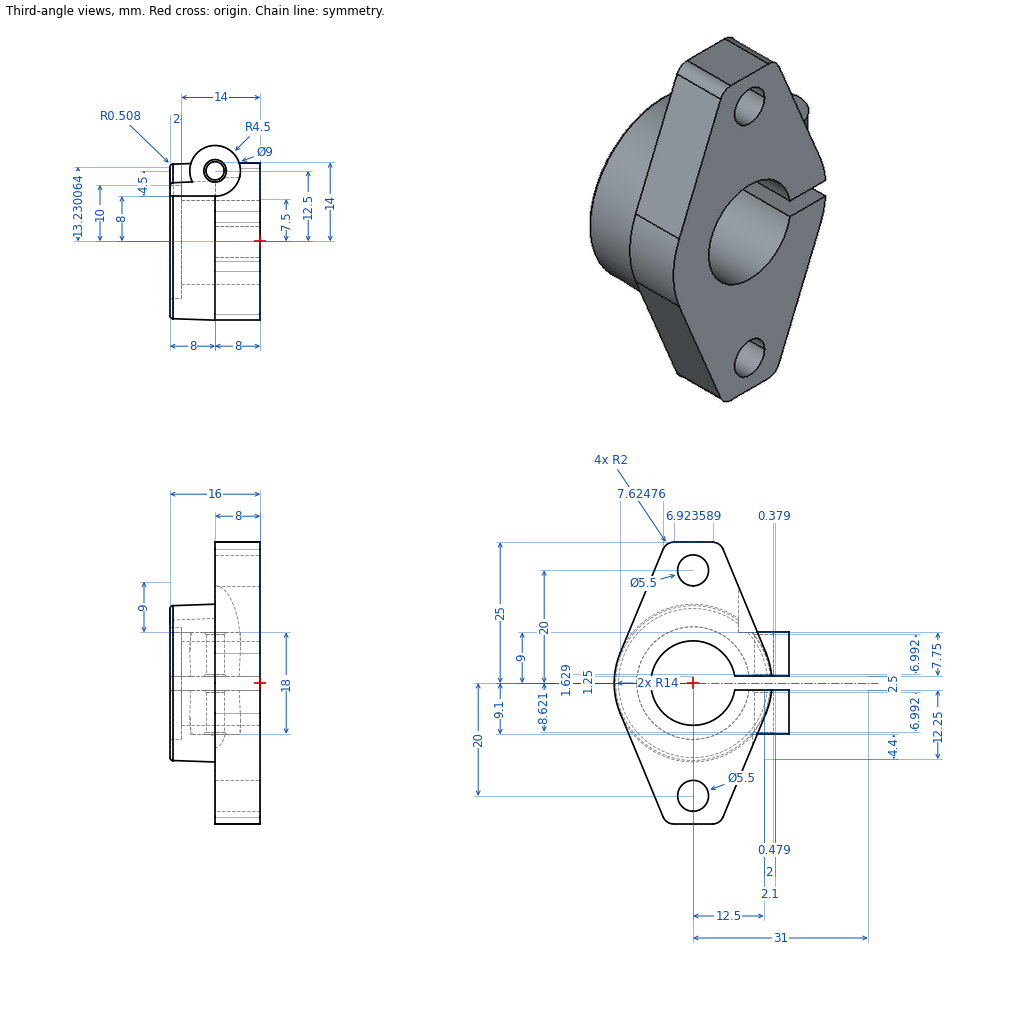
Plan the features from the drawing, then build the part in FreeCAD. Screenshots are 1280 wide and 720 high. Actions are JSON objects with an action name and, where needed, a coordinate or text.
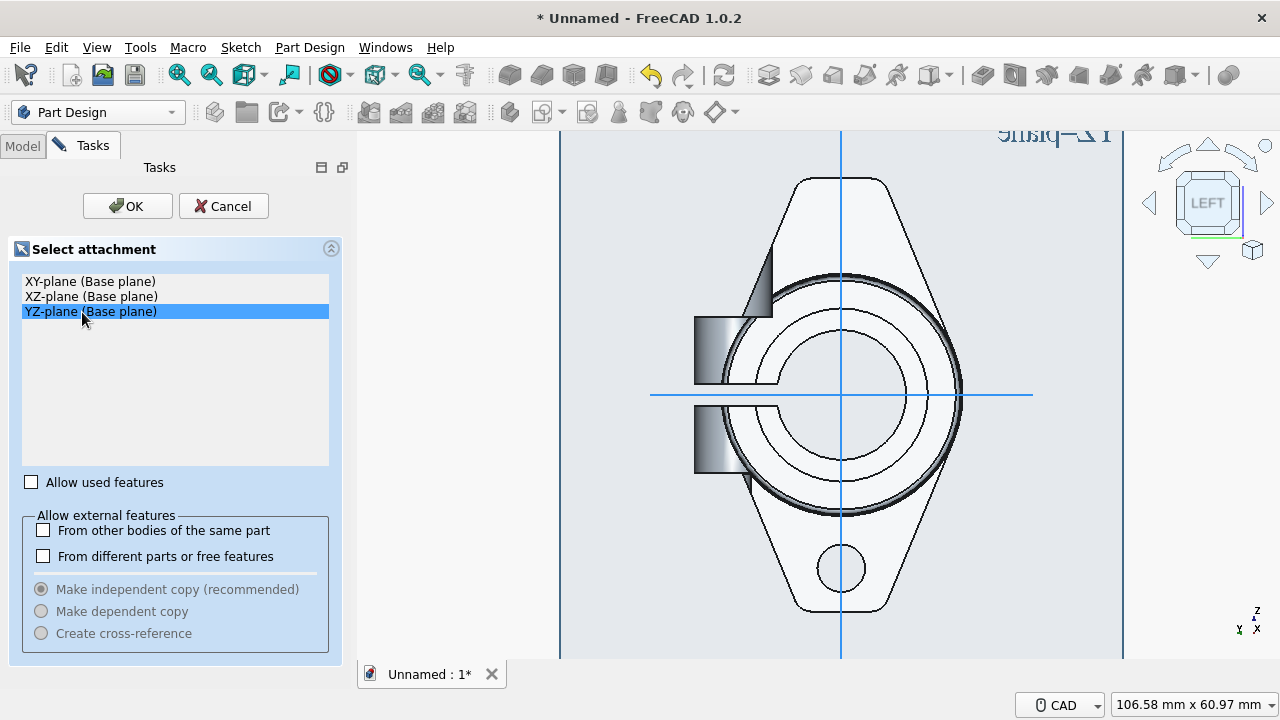
{"action": "left_click", "coordinate": [128, 206]}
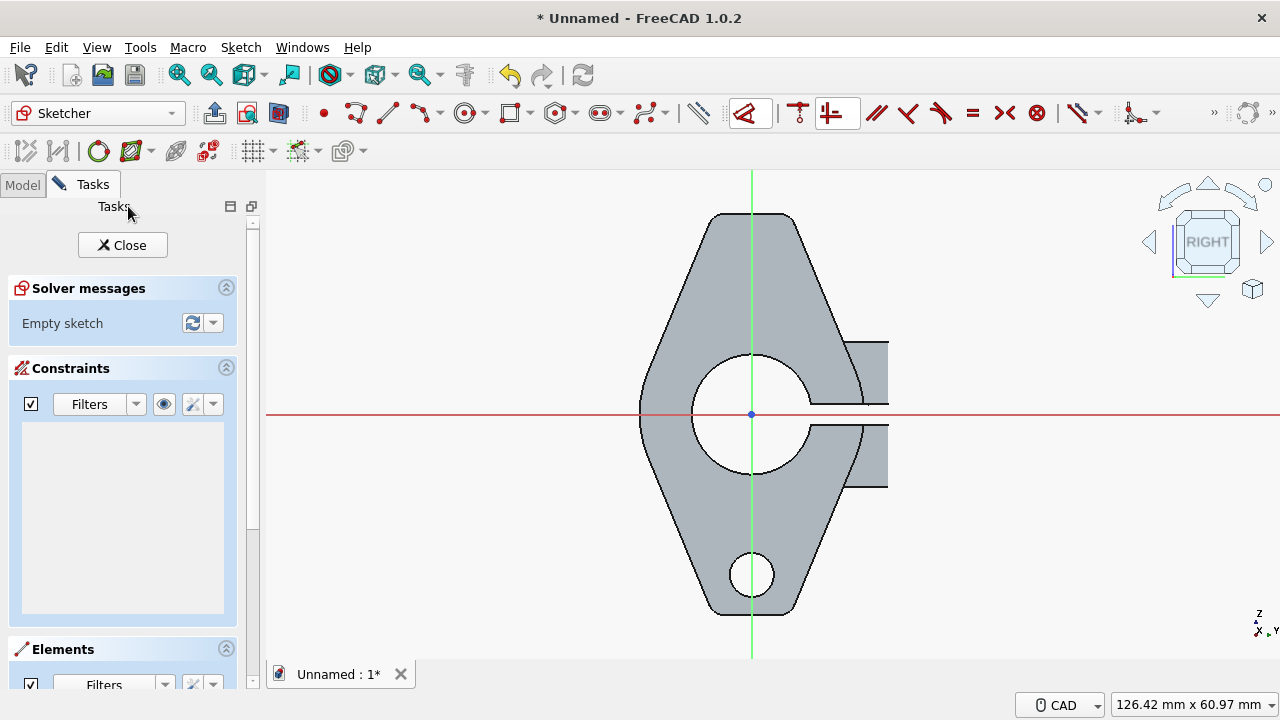
{"action": "scroll", "coordinate": [759, 229], "scroll_direction": "up", "scroll_amount": 10}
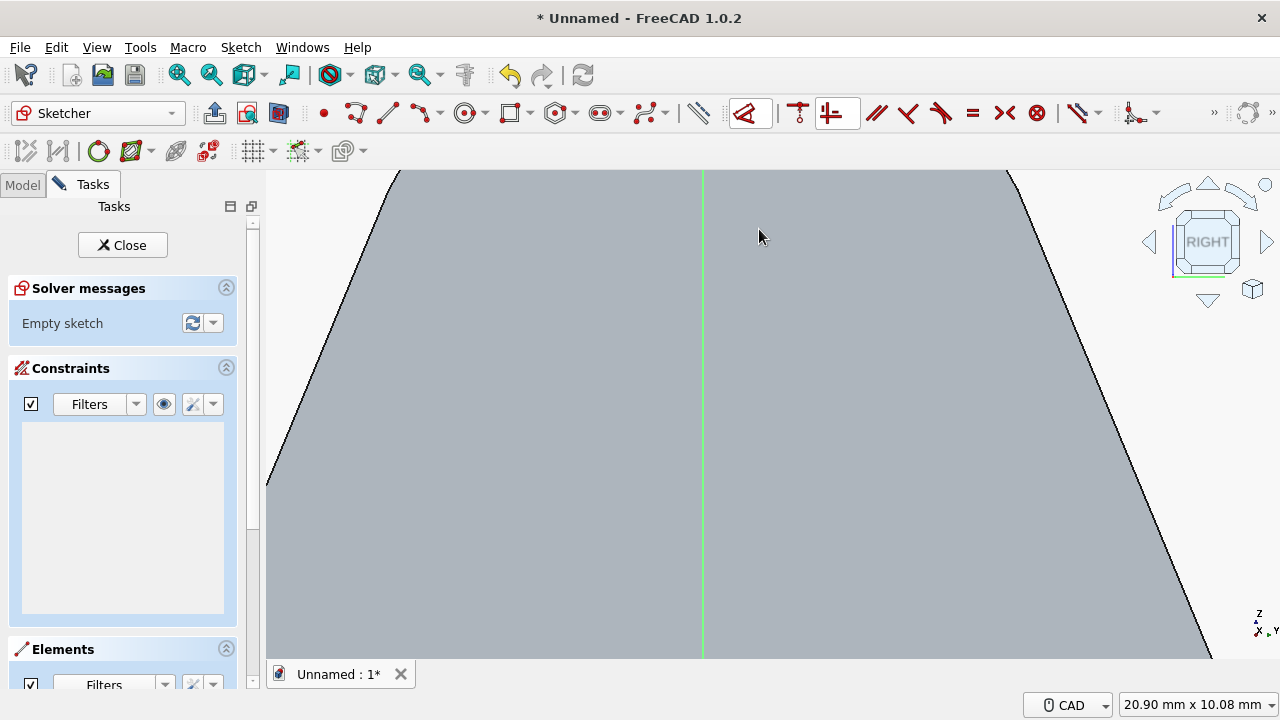
{"action": "left_click", "coordinate": [466, 114]}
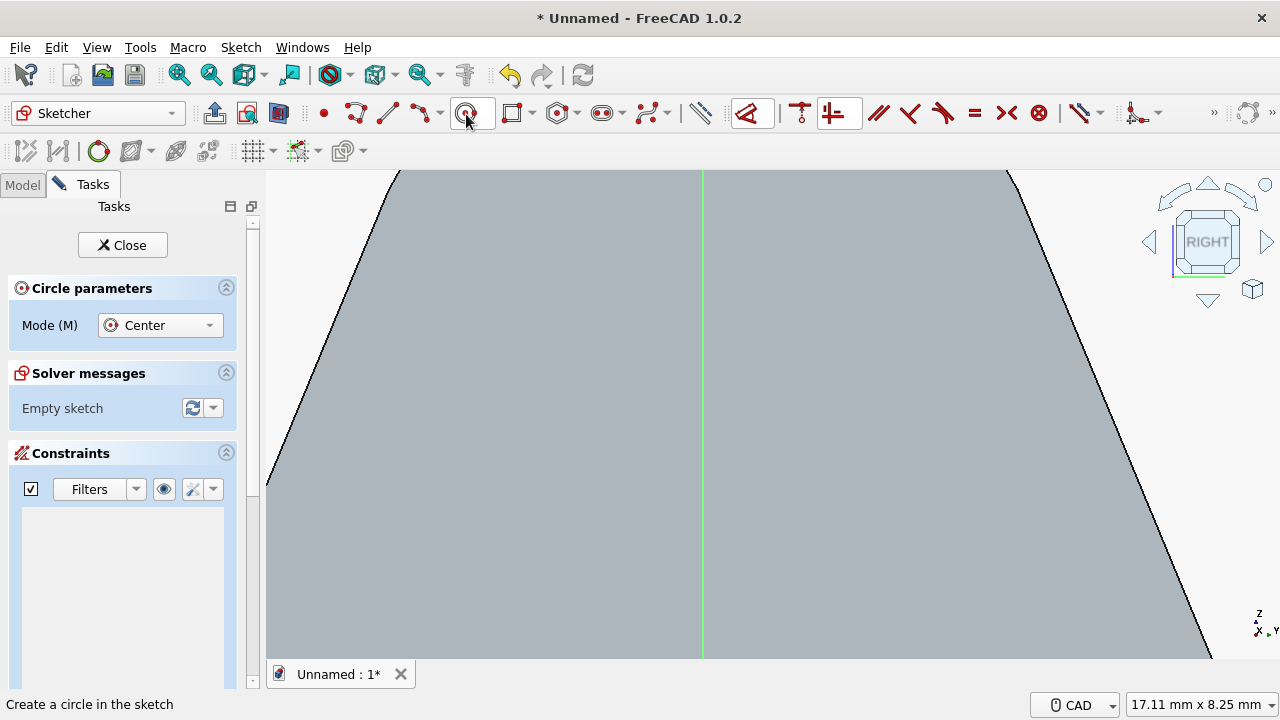
{"action": "left_click", "coordinate": [703, 414]}
{"action": "mouse_move", "coordinate": [818, 298]}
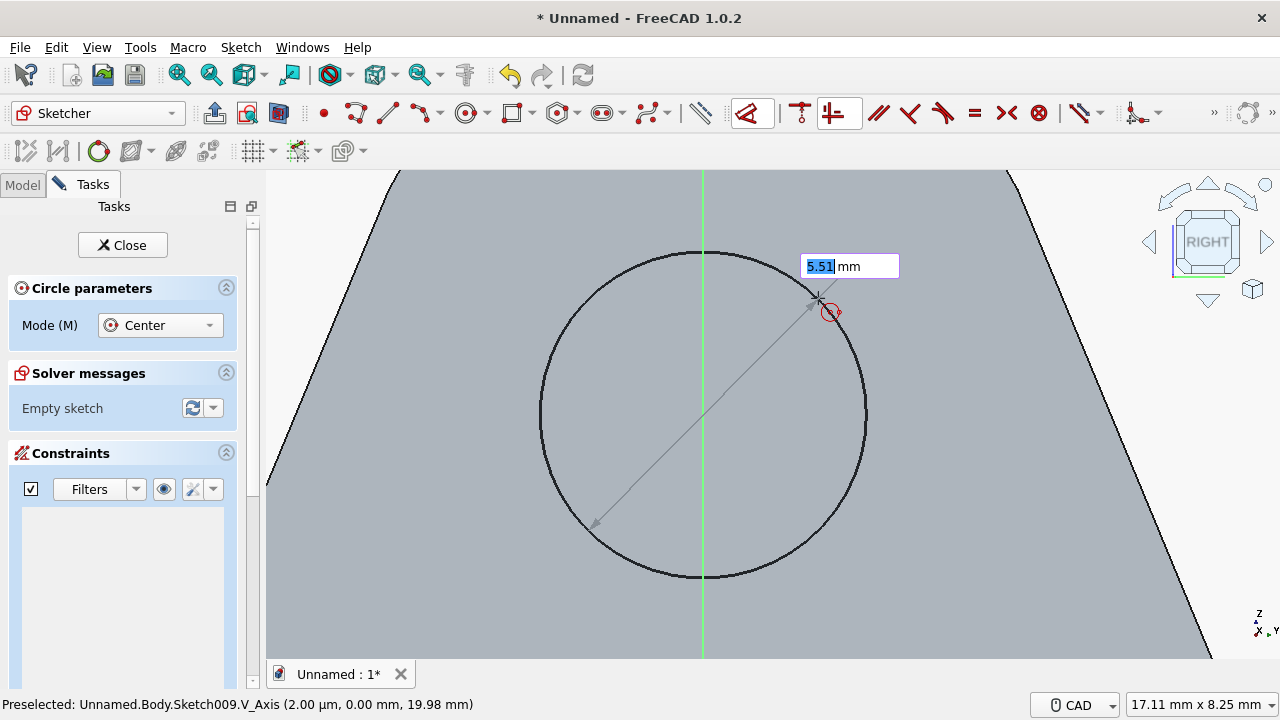
{"action": "type", "text": "5.5"}
{"action": "key", "text": "Return"}
{"action": "key", "text": "Escape"}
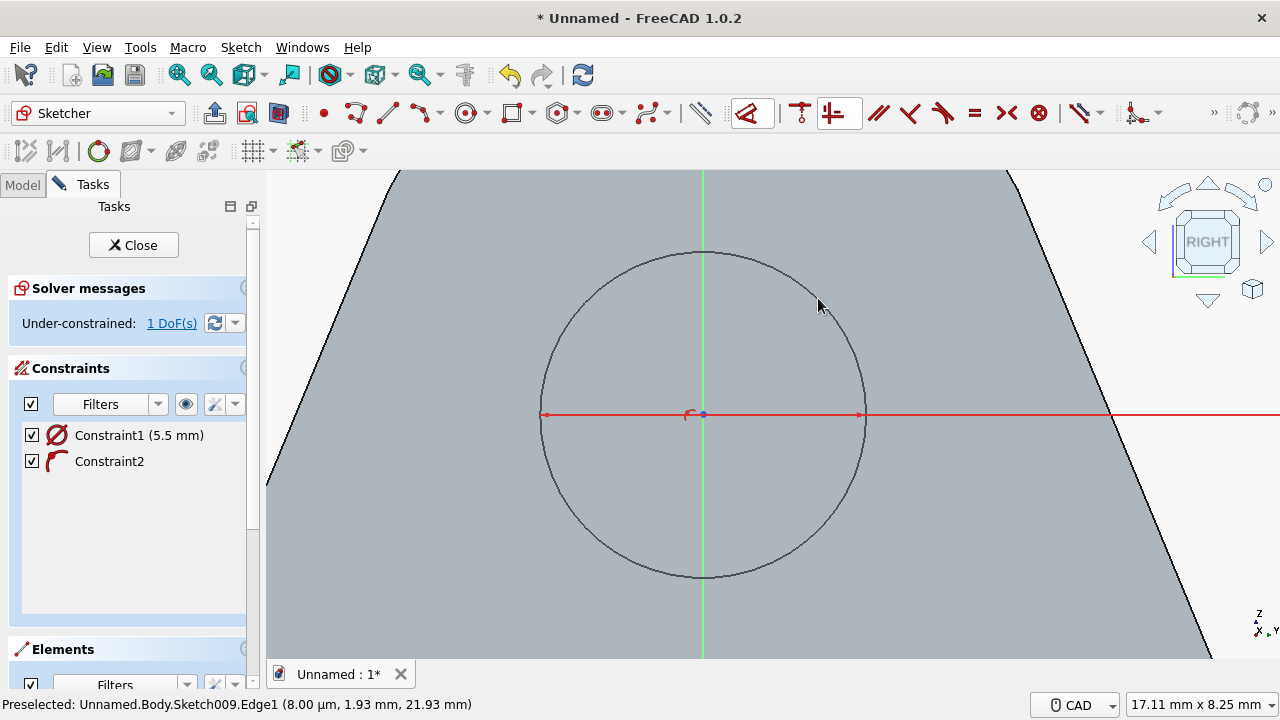
{"action": "left_click", "coordinate": [703, 415]}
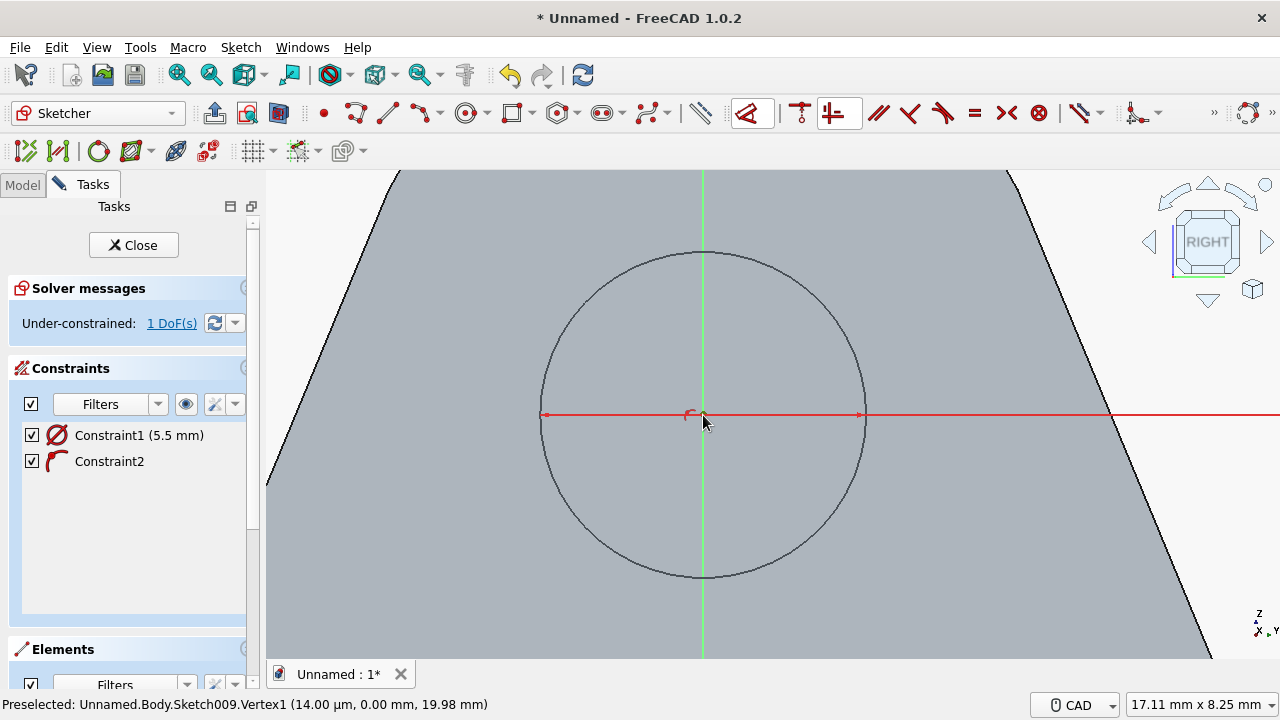
{"action": "left_click", "coordinate": [768, 114]}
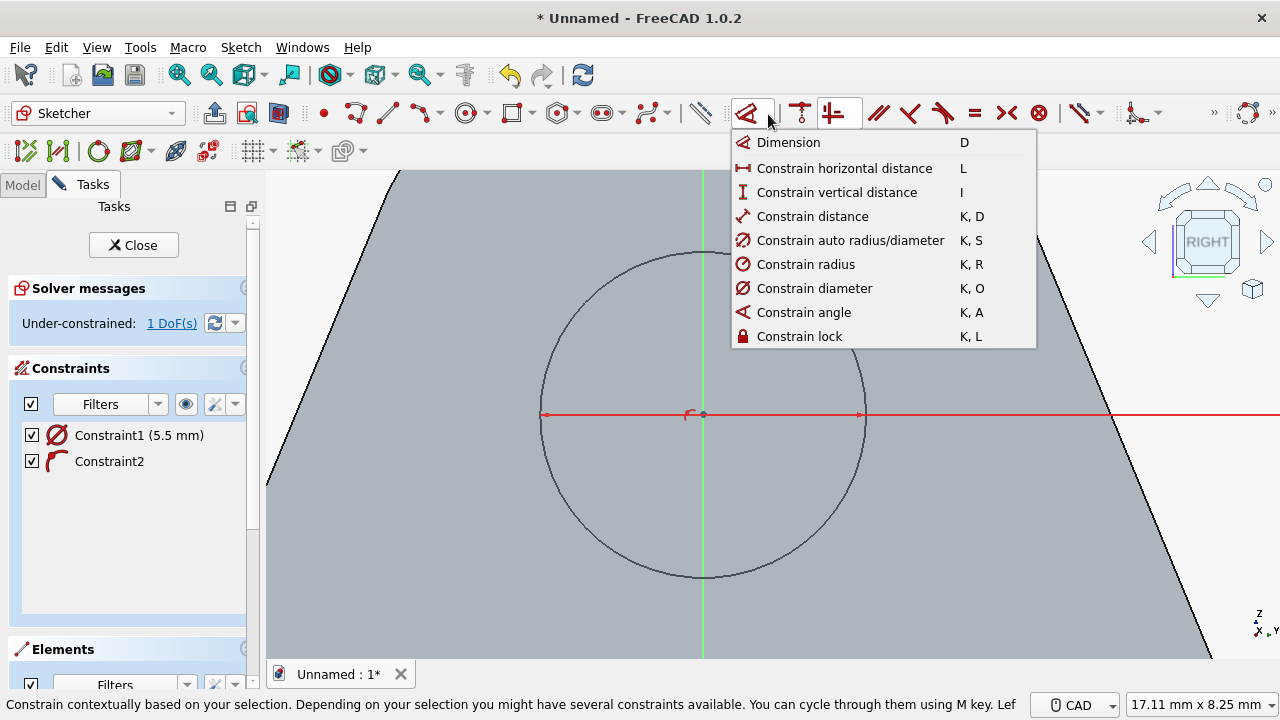
{"action": "left_click", "coordinate": [884, 192]}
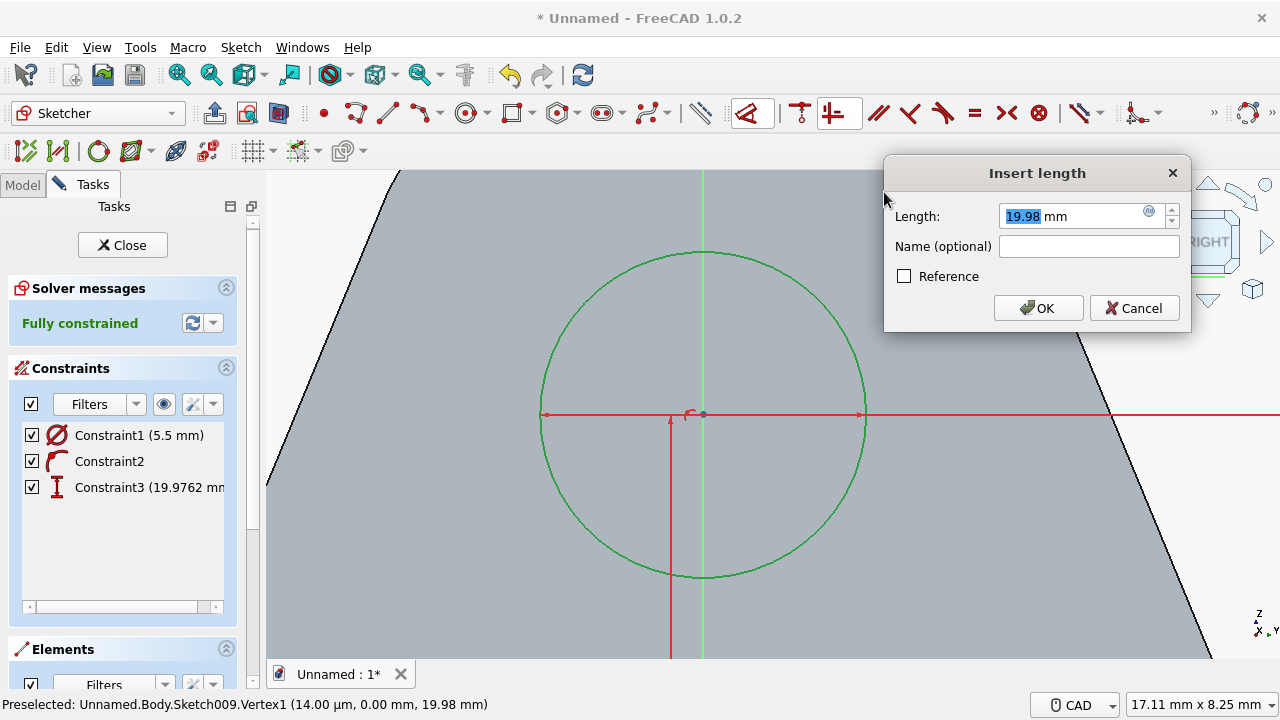
{"action": "type", "text": "20"}
{"action": "key", "text": "Return"}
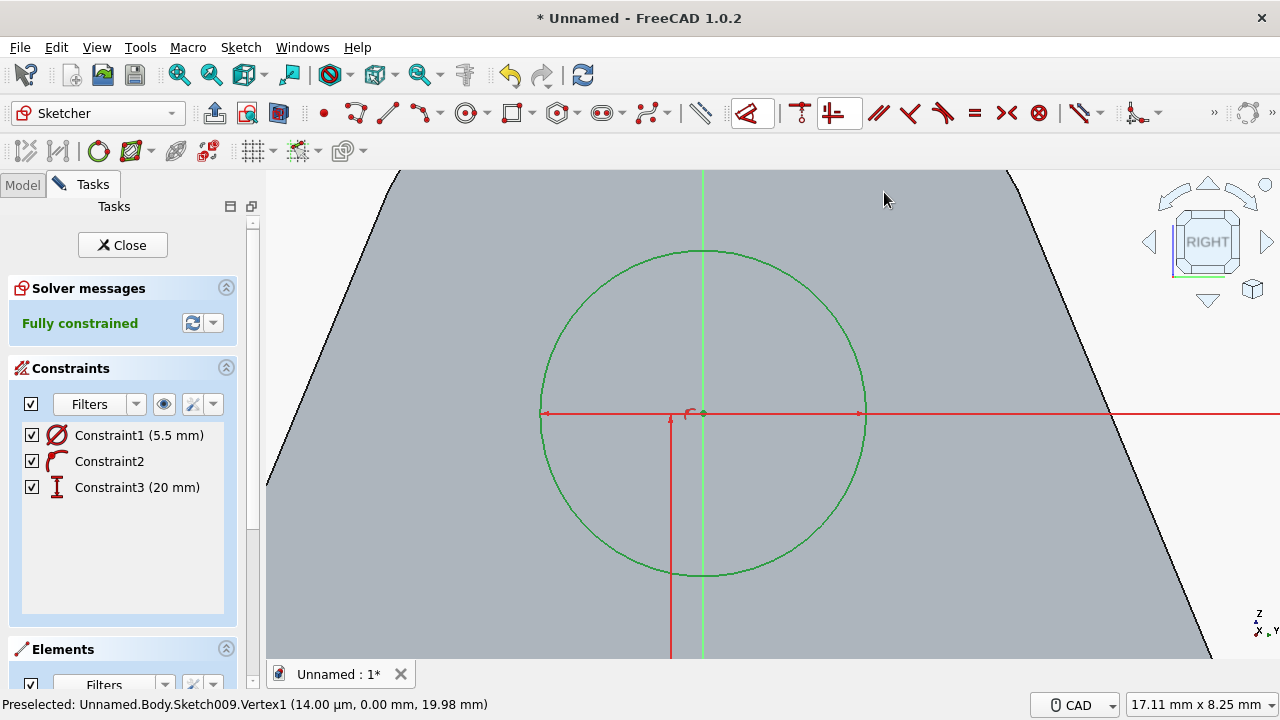
{"action": "left_click", "coordinate": [123, 245]}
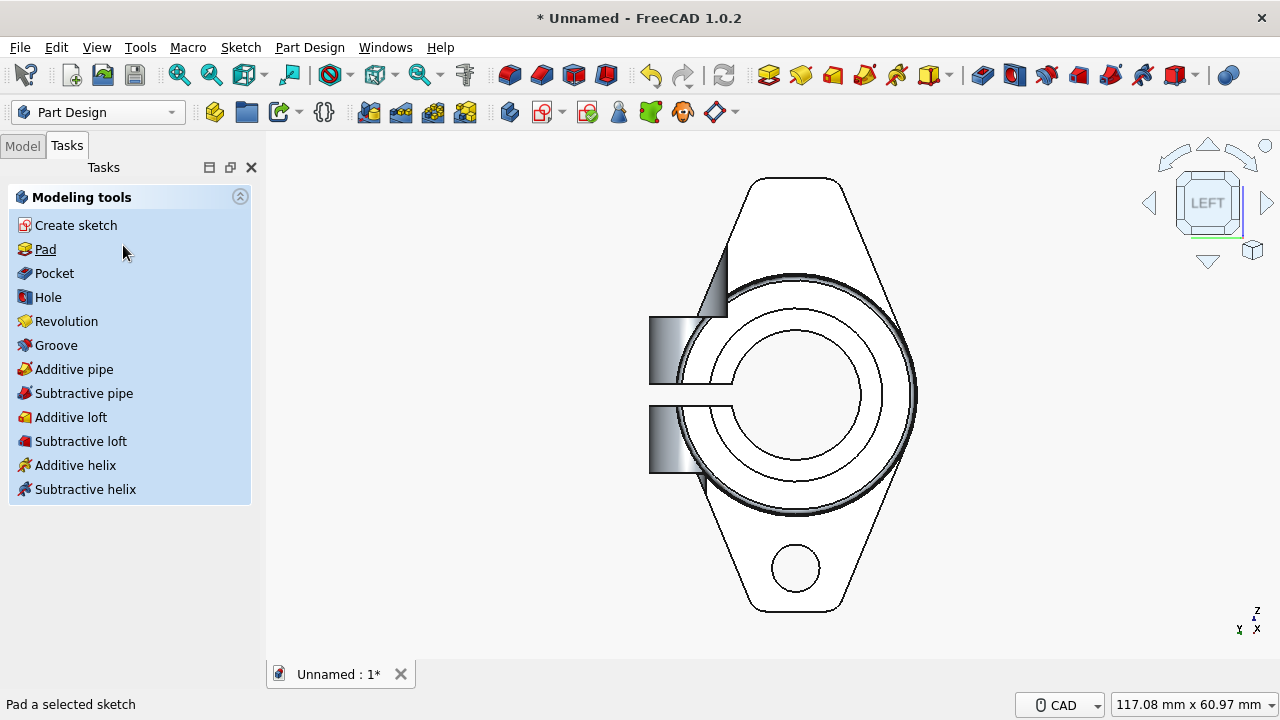
{"action": "left_click", "coordinate": [984, 76]}